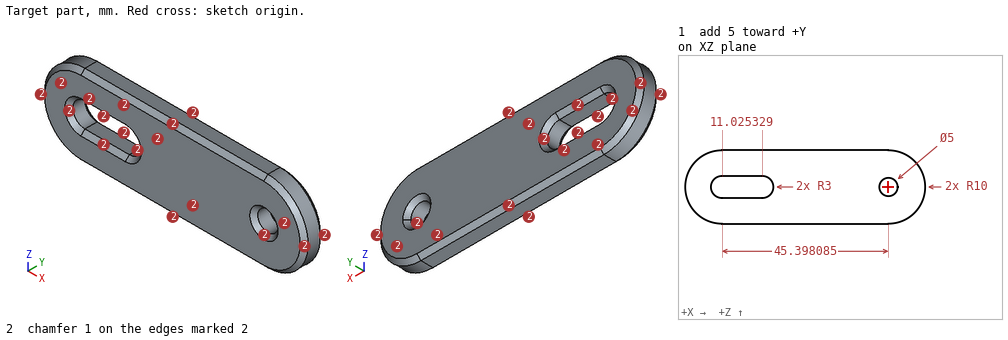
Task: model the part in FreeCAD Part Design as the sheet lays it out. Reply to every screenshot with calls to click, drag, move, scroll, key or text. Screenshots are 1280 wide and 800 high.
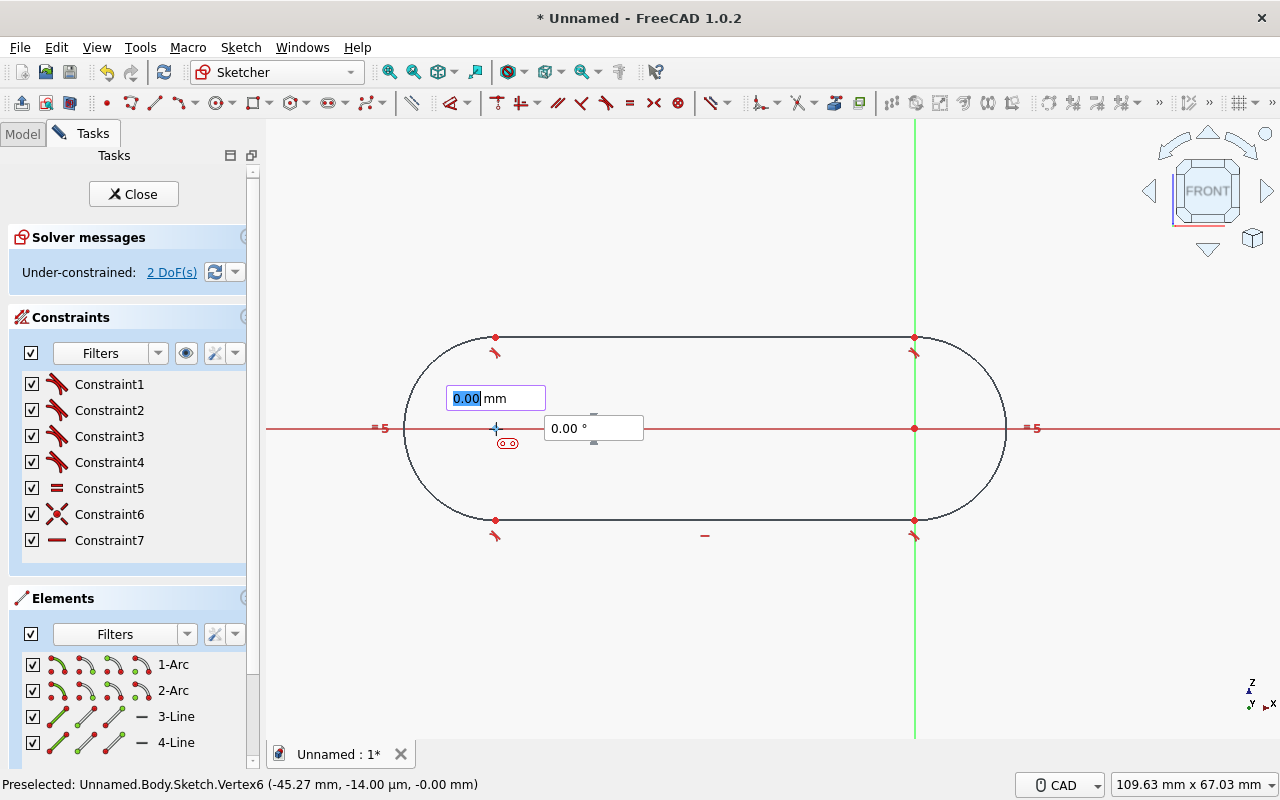
click(597, 411)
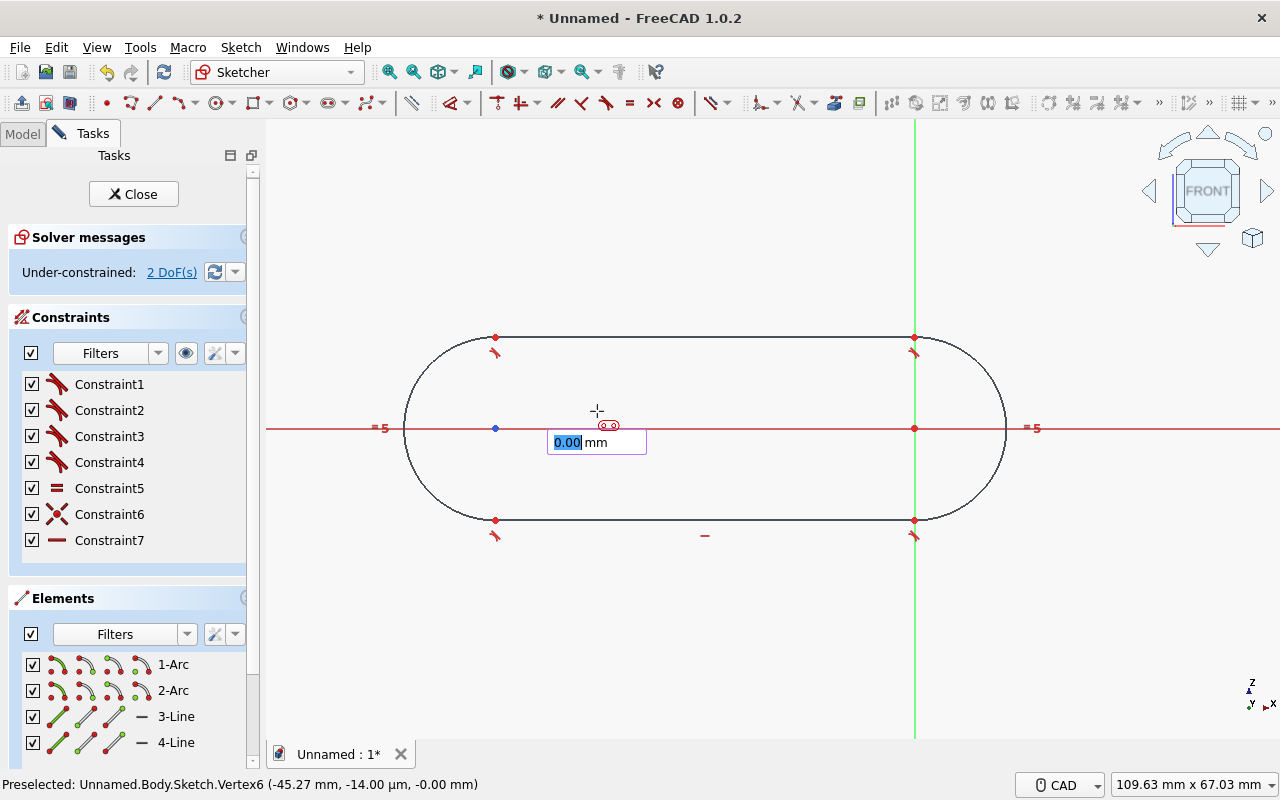
click(546, 457)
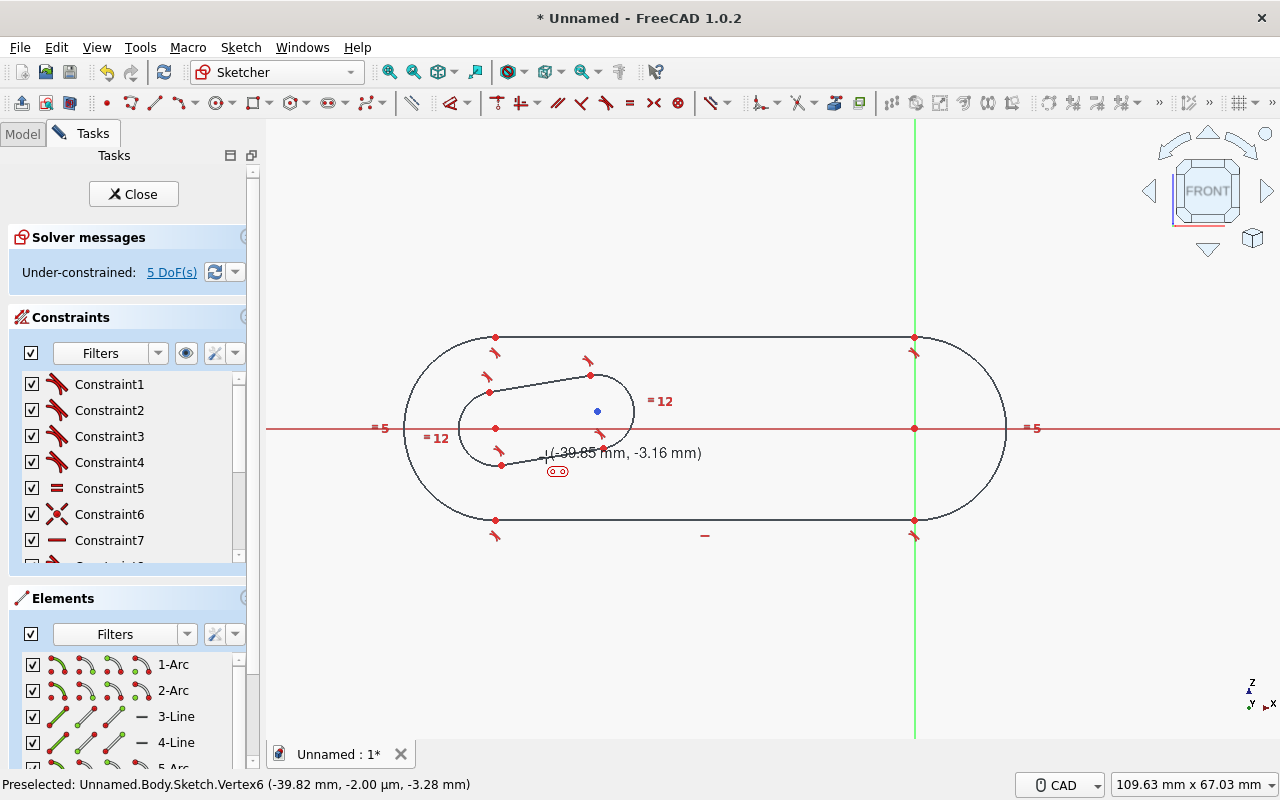
click(216, 104)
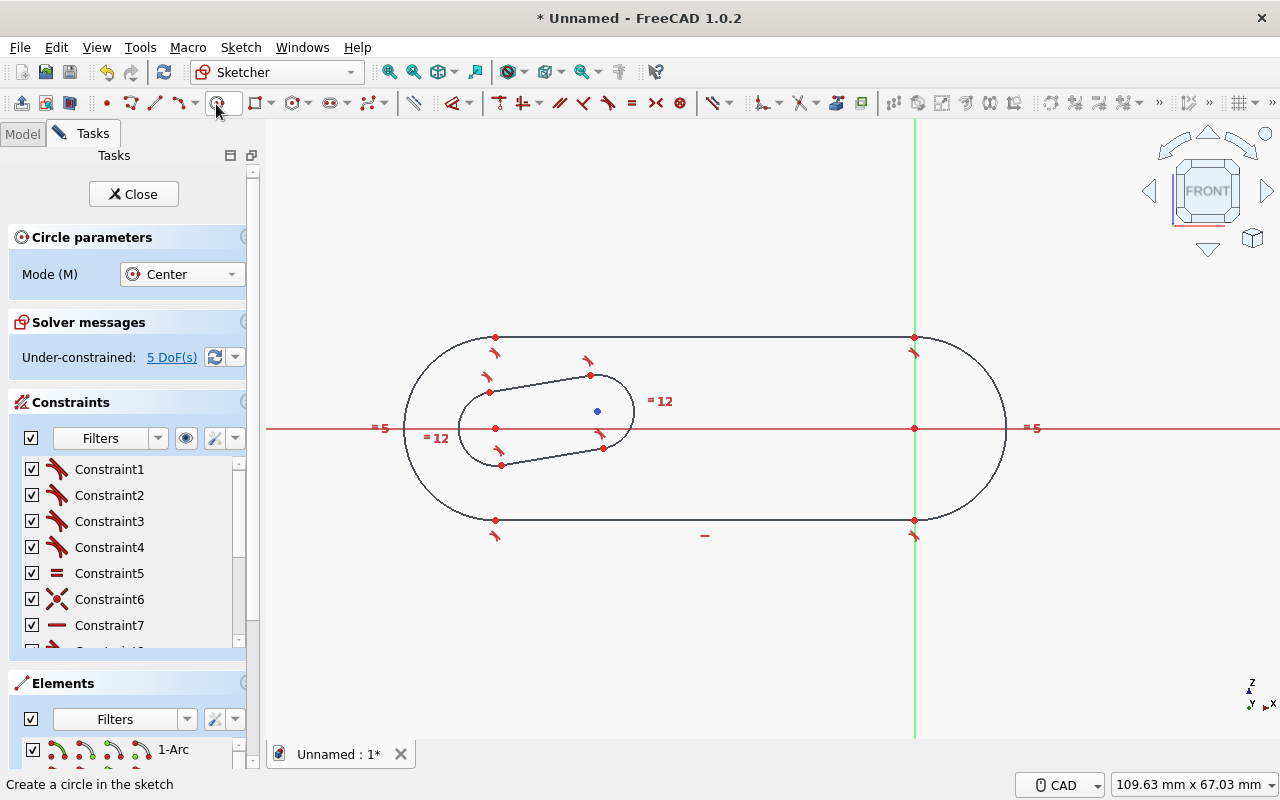
click(915, 429)
move(931, 412)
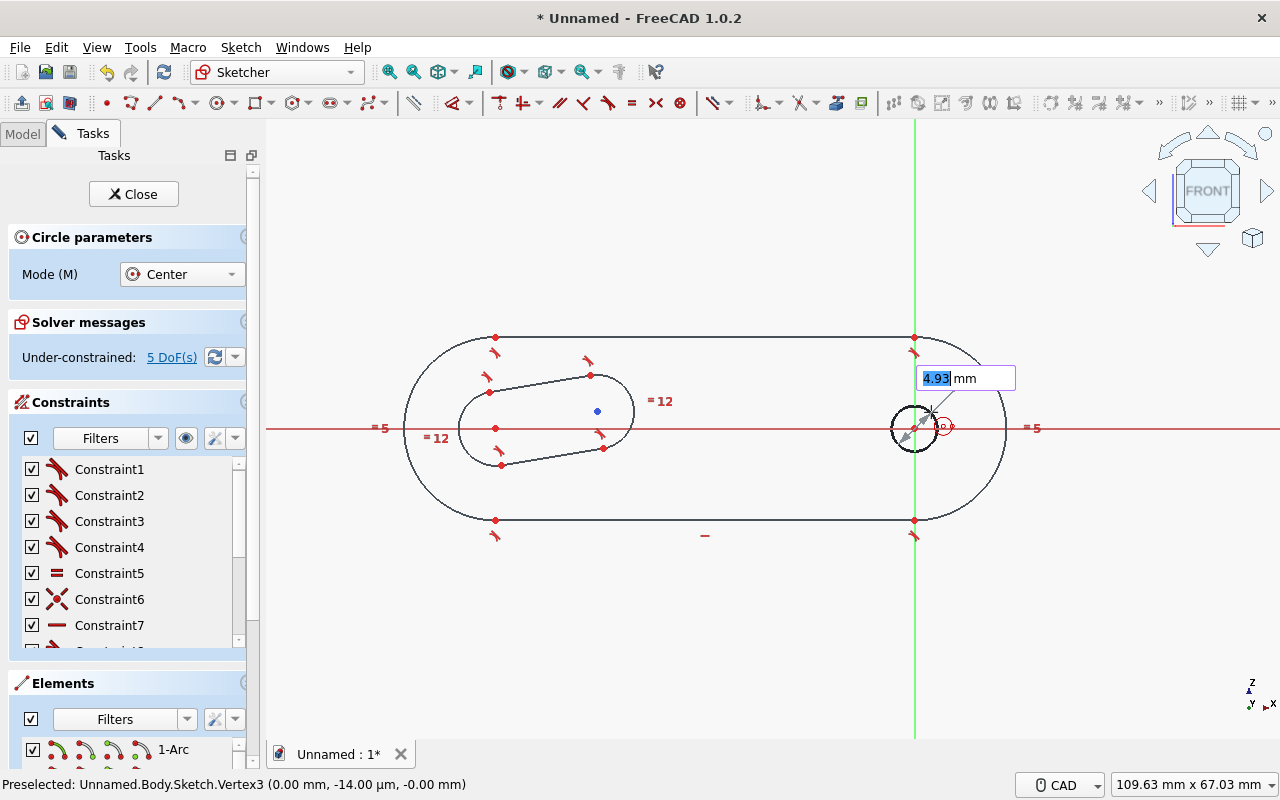
text(5)
key(Return)
key(Escape)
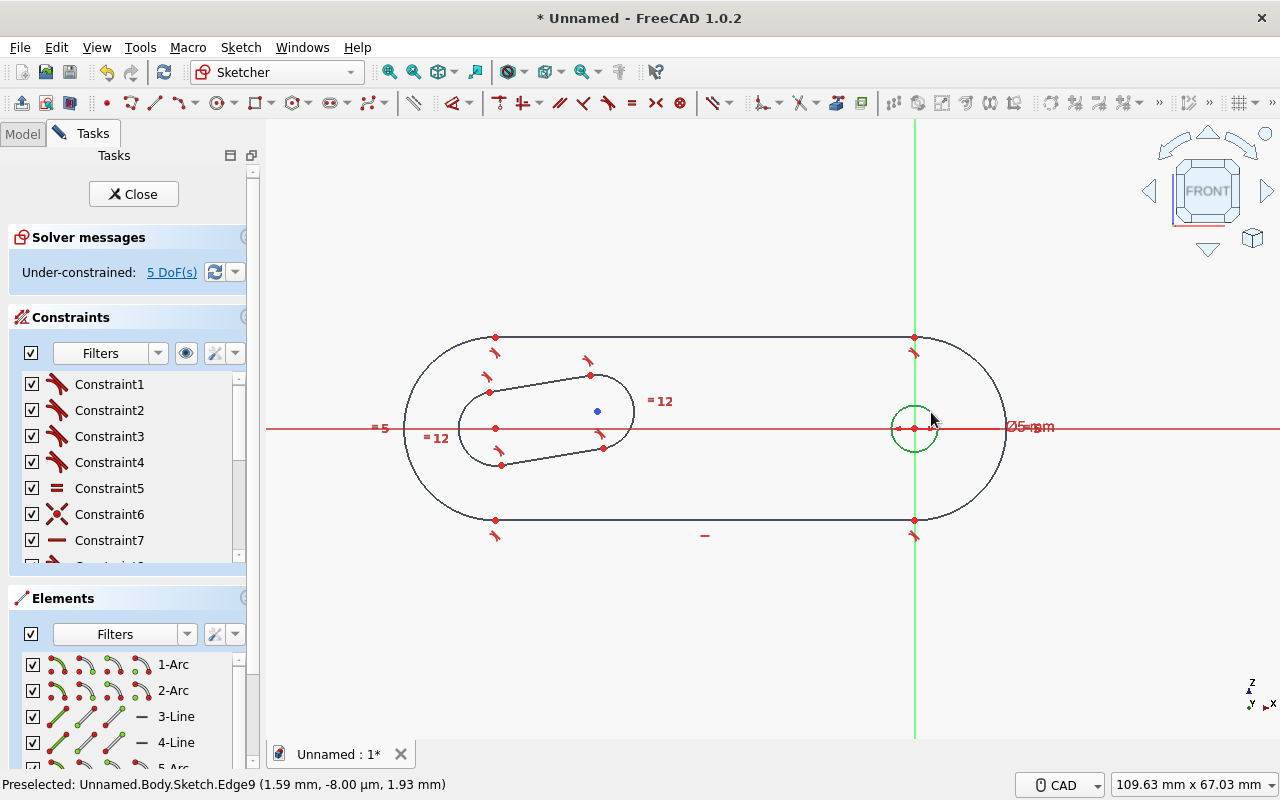
click(520, 387)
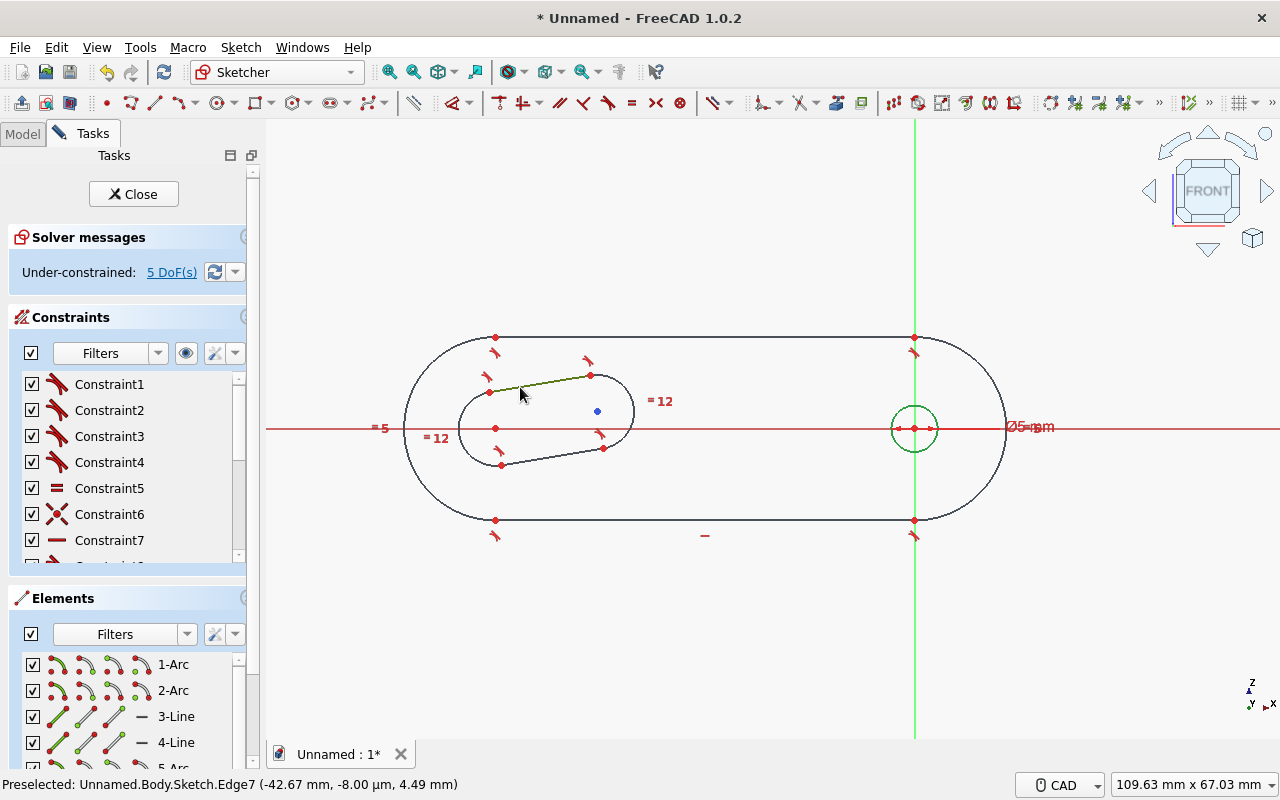
key(h)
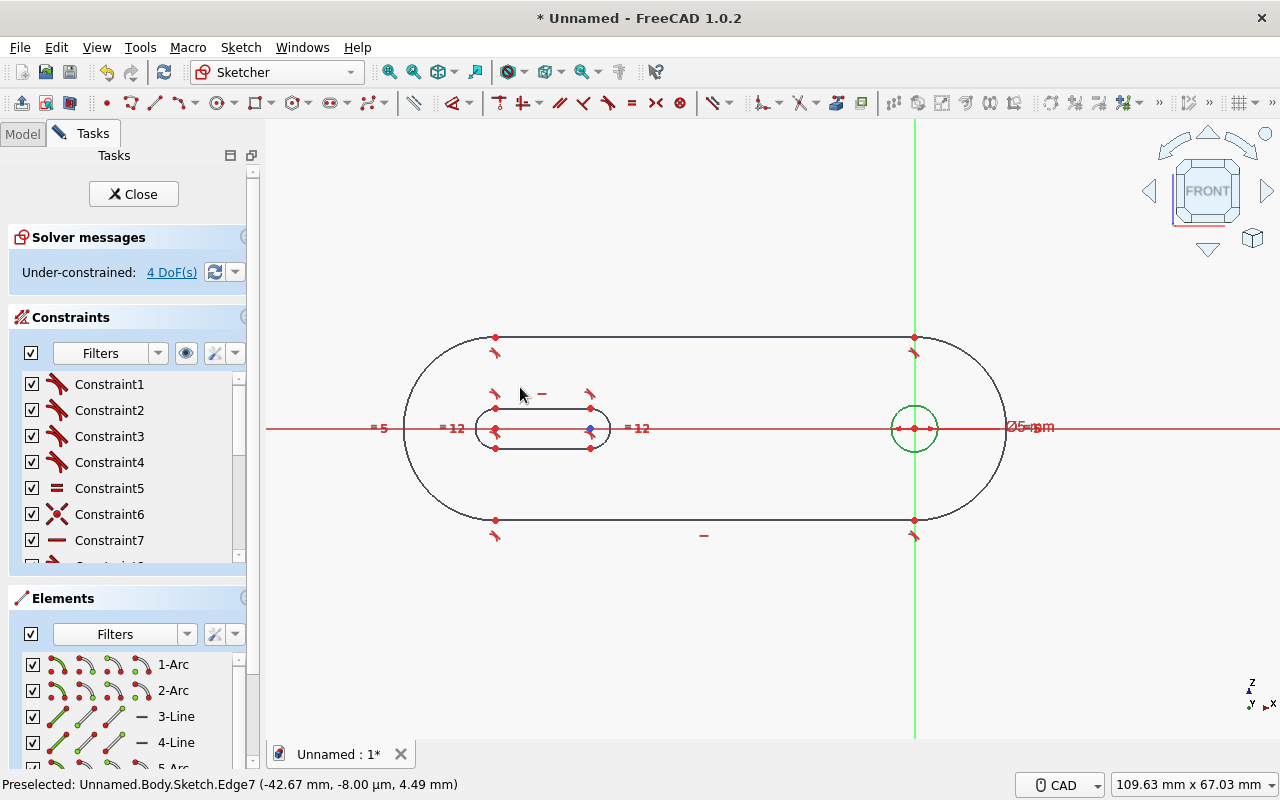
click(452, 104)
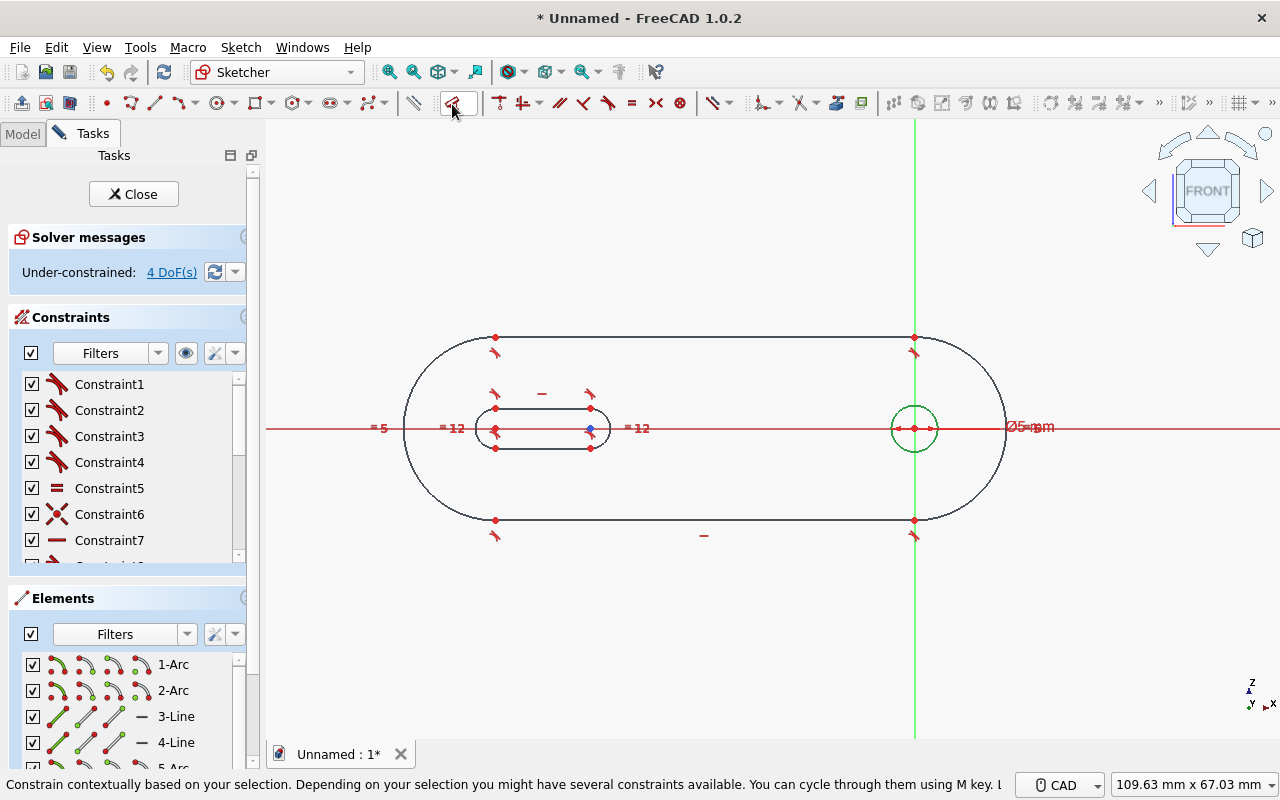
click(989, 483)
click(1015, 502)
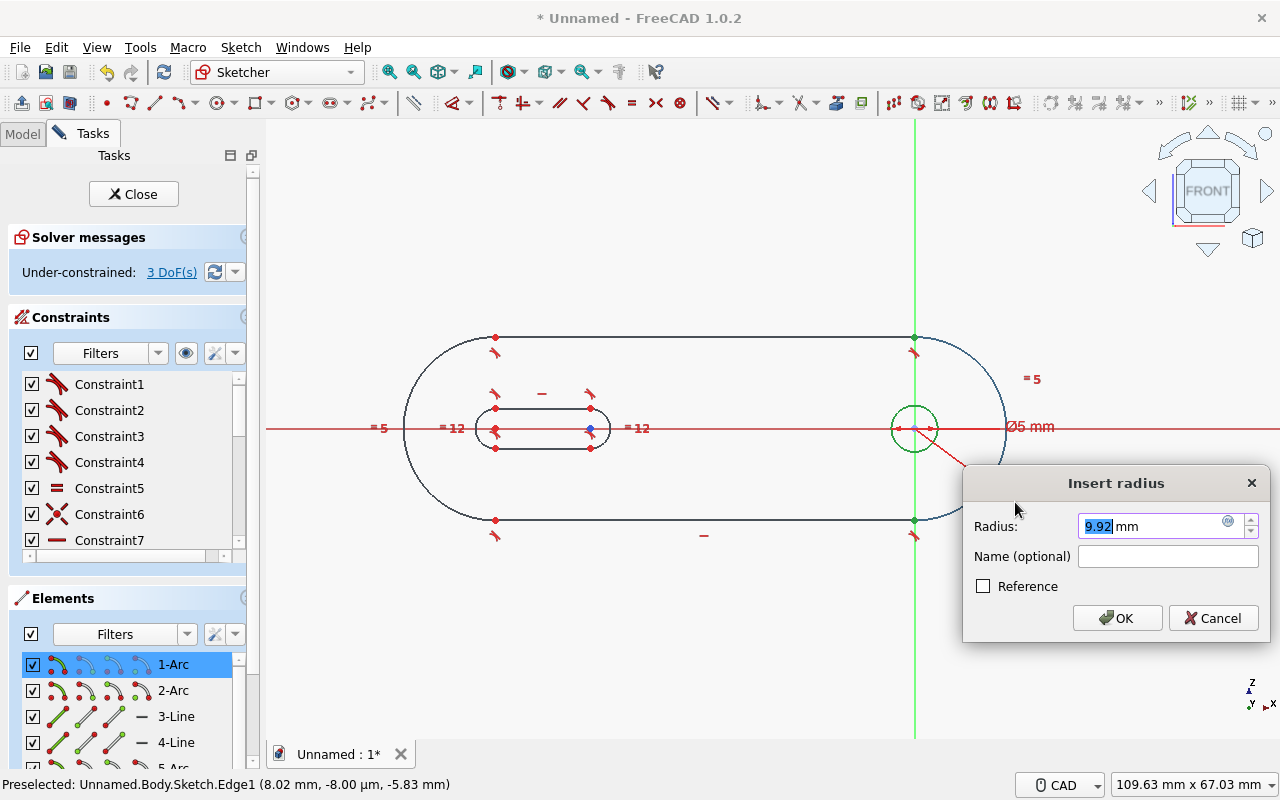
text(10)
key(Return)